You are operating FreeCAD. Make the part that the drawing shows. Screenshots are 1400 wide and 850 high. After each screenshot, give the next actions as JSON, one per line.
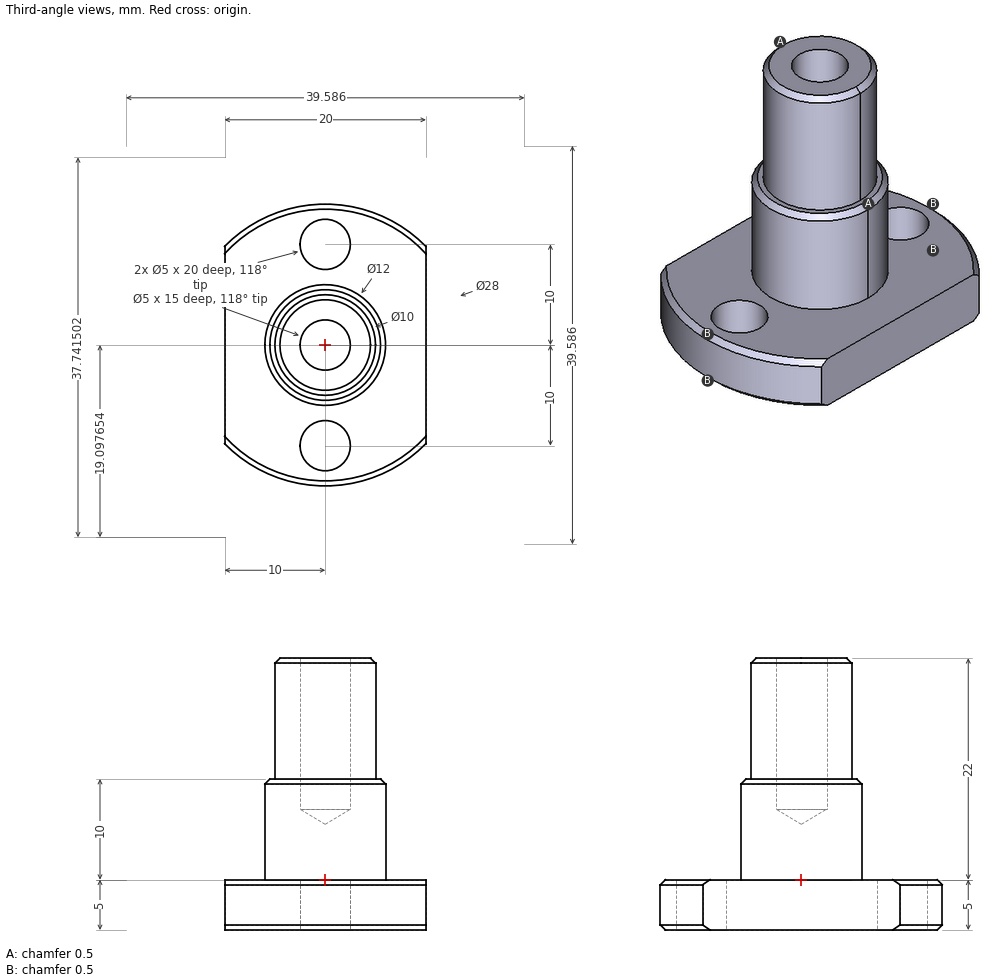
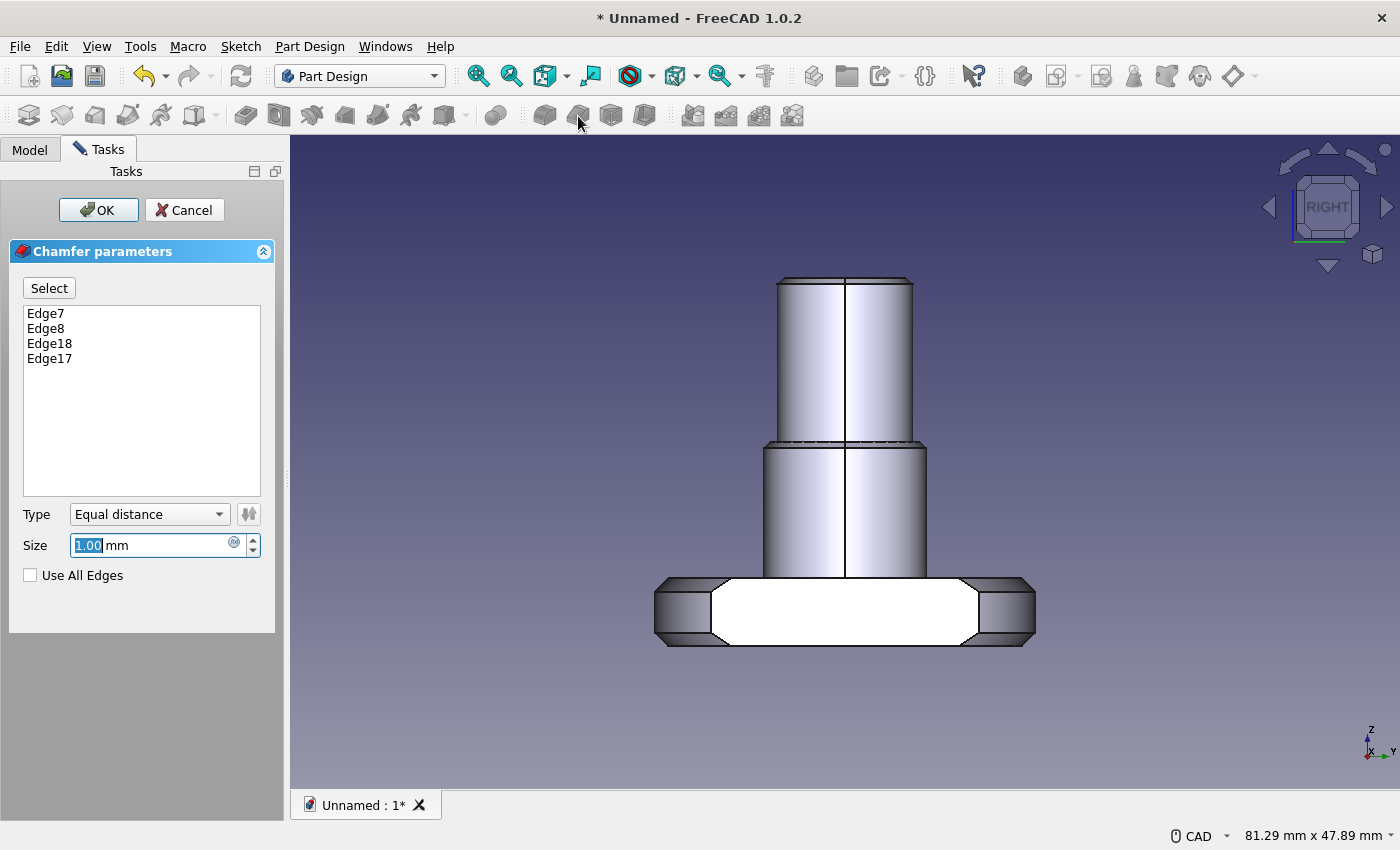
{"action": "type", "text": "0.5"}
{"action": "key", "text": "Tab"}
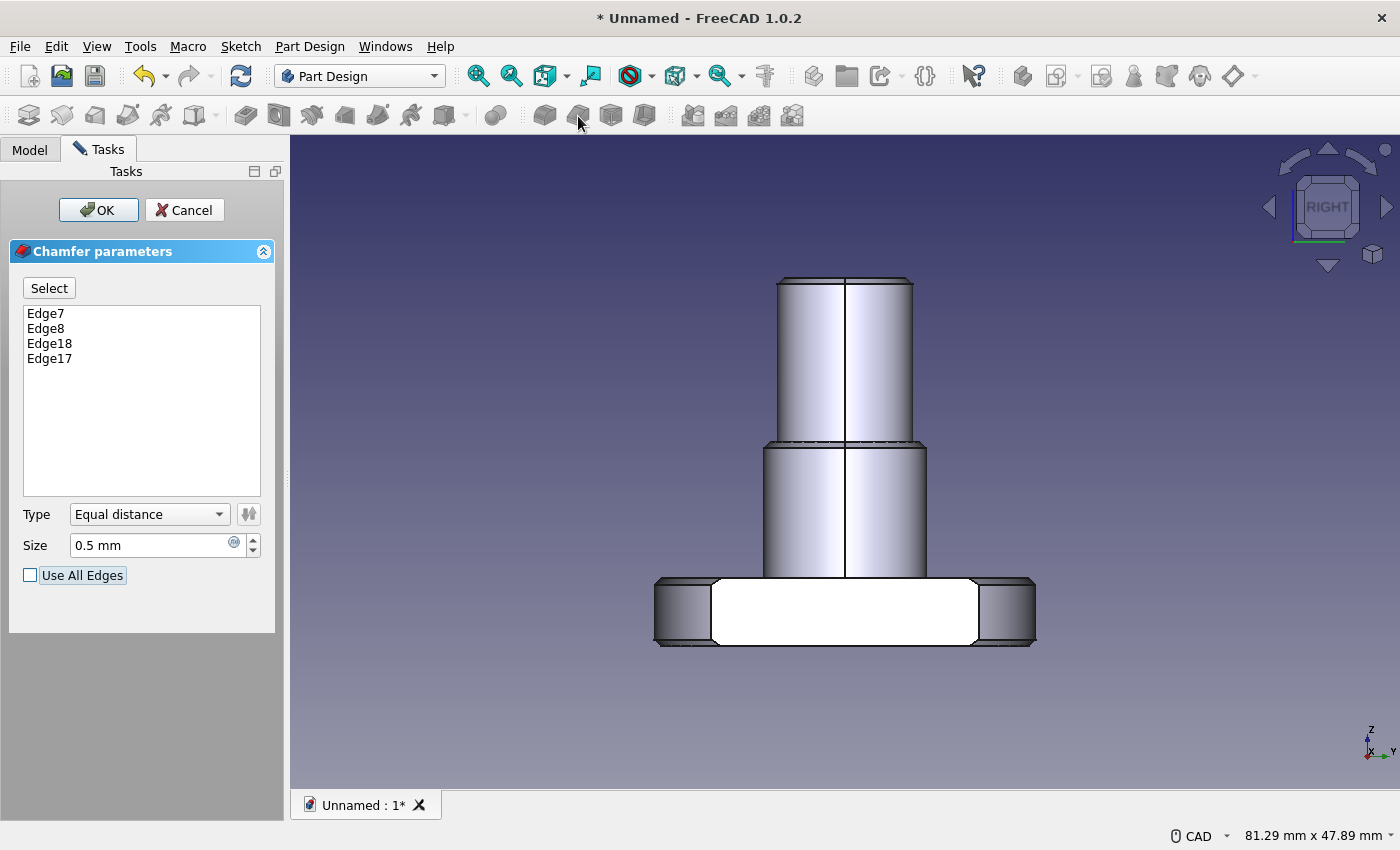
{"action": "left_click", "coordinate": [99, 210]}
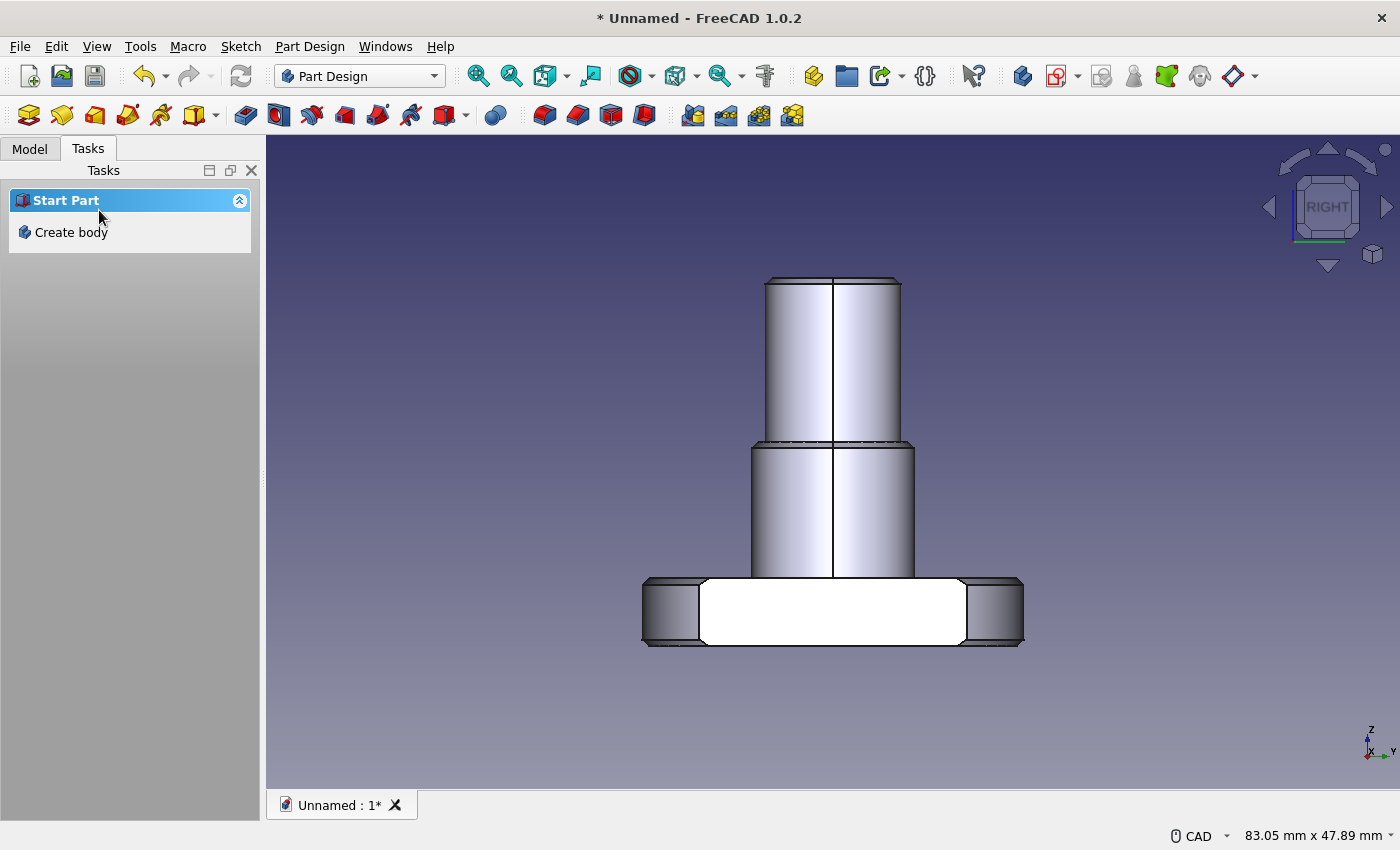
{"action": "key", "text": "0"}